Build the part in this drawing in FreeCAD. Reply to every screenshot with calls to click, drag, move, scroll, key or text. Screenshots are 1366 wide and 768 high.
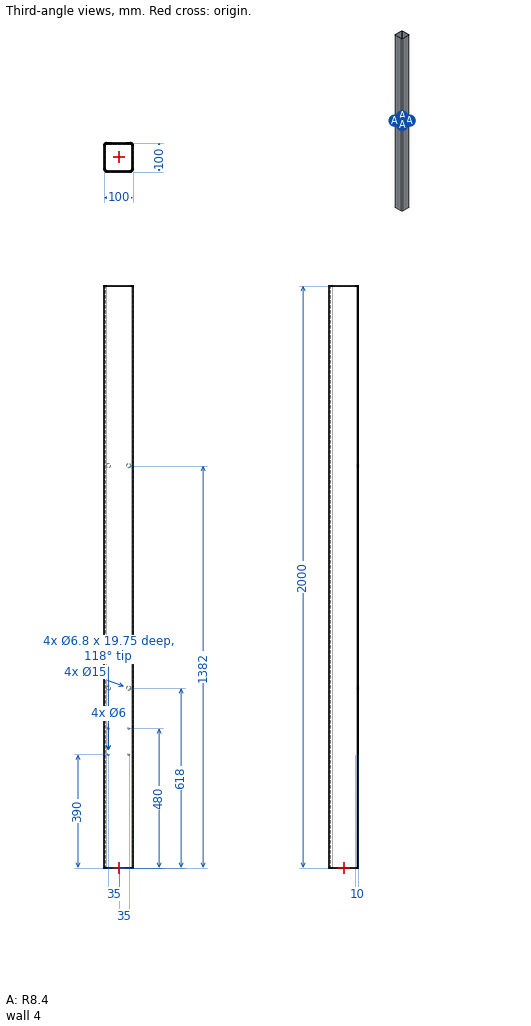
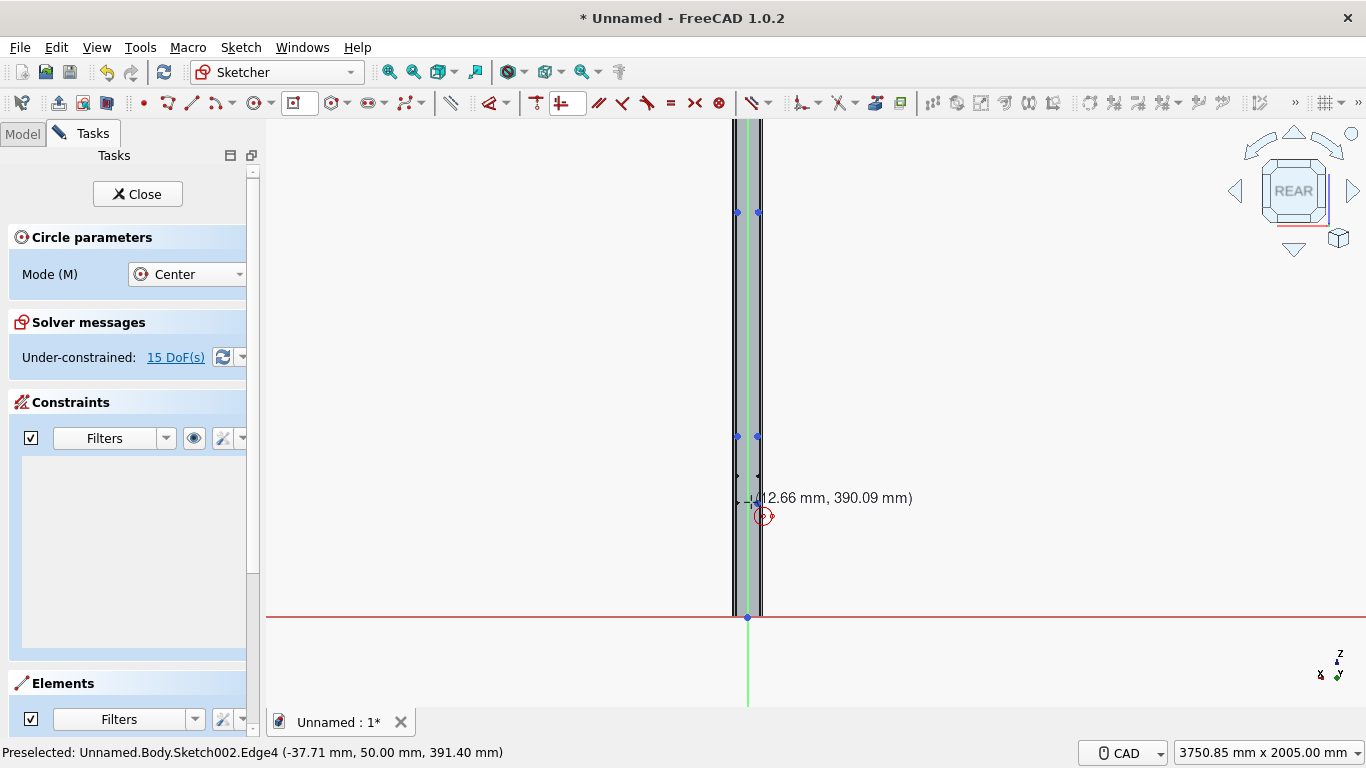
scroll(737, 503, up, 3)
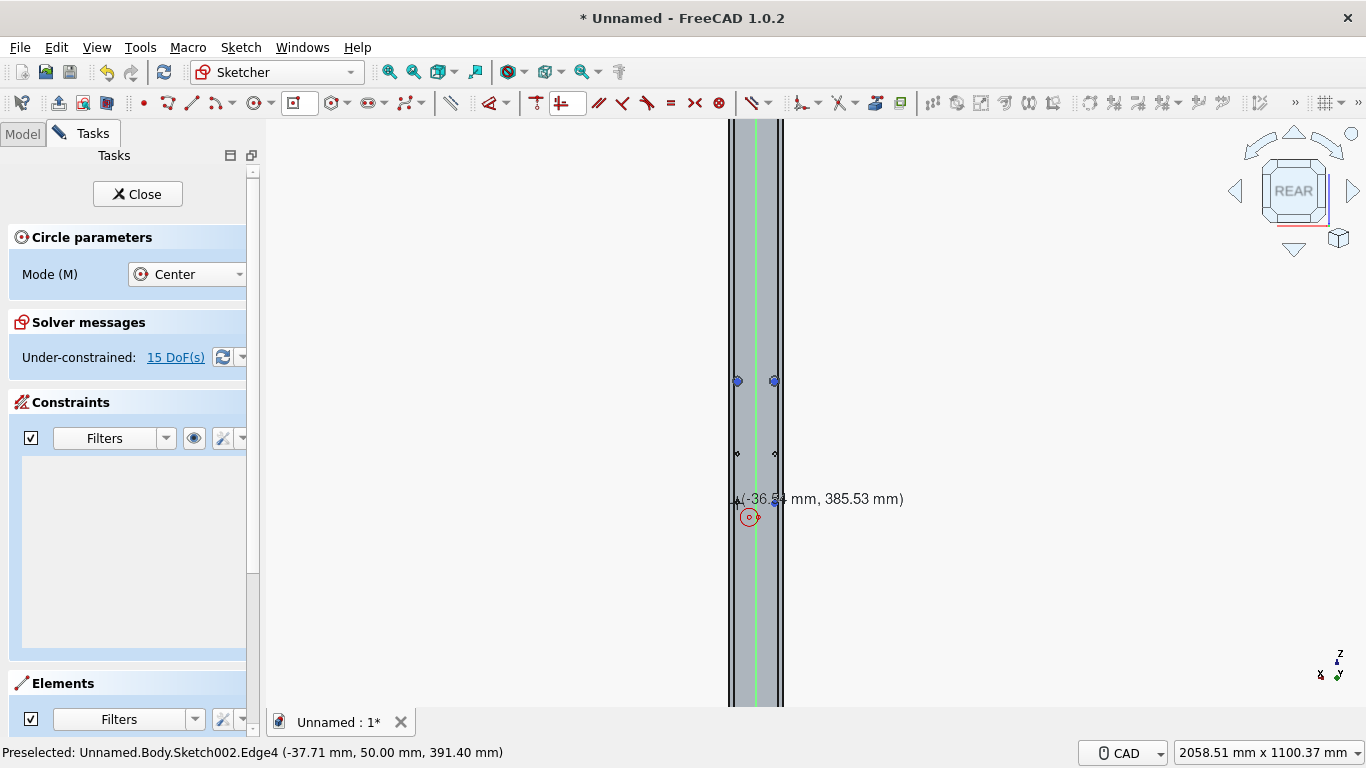
click(737, 502)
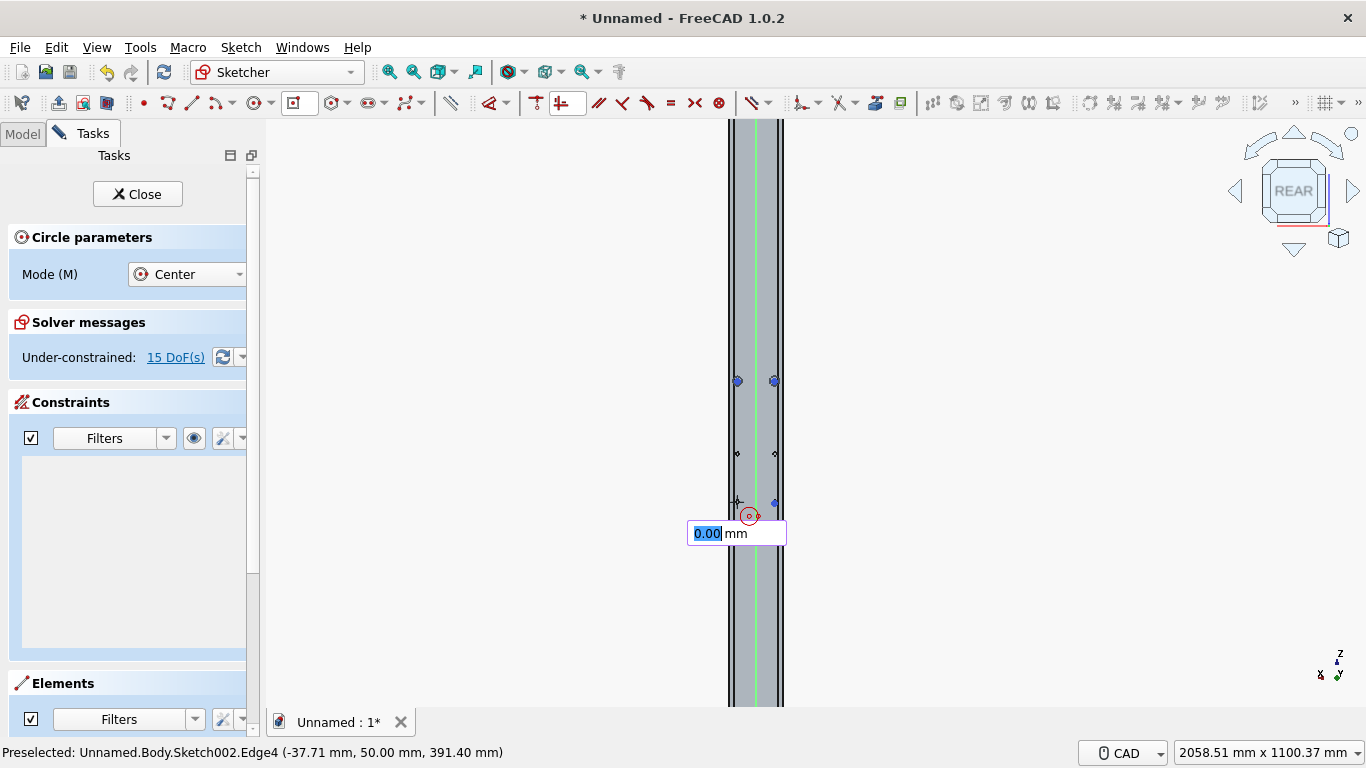
scroll(739, 501, up, 12)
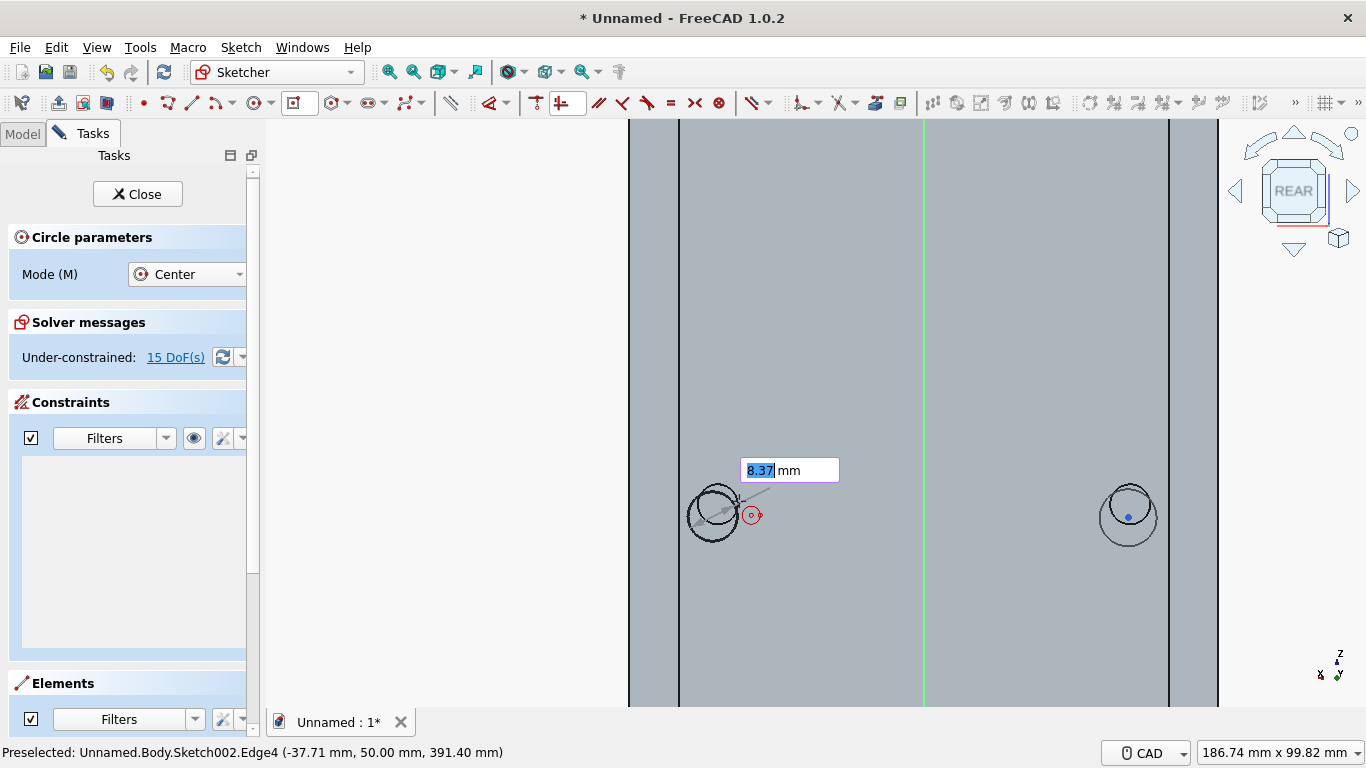
click(730, 492)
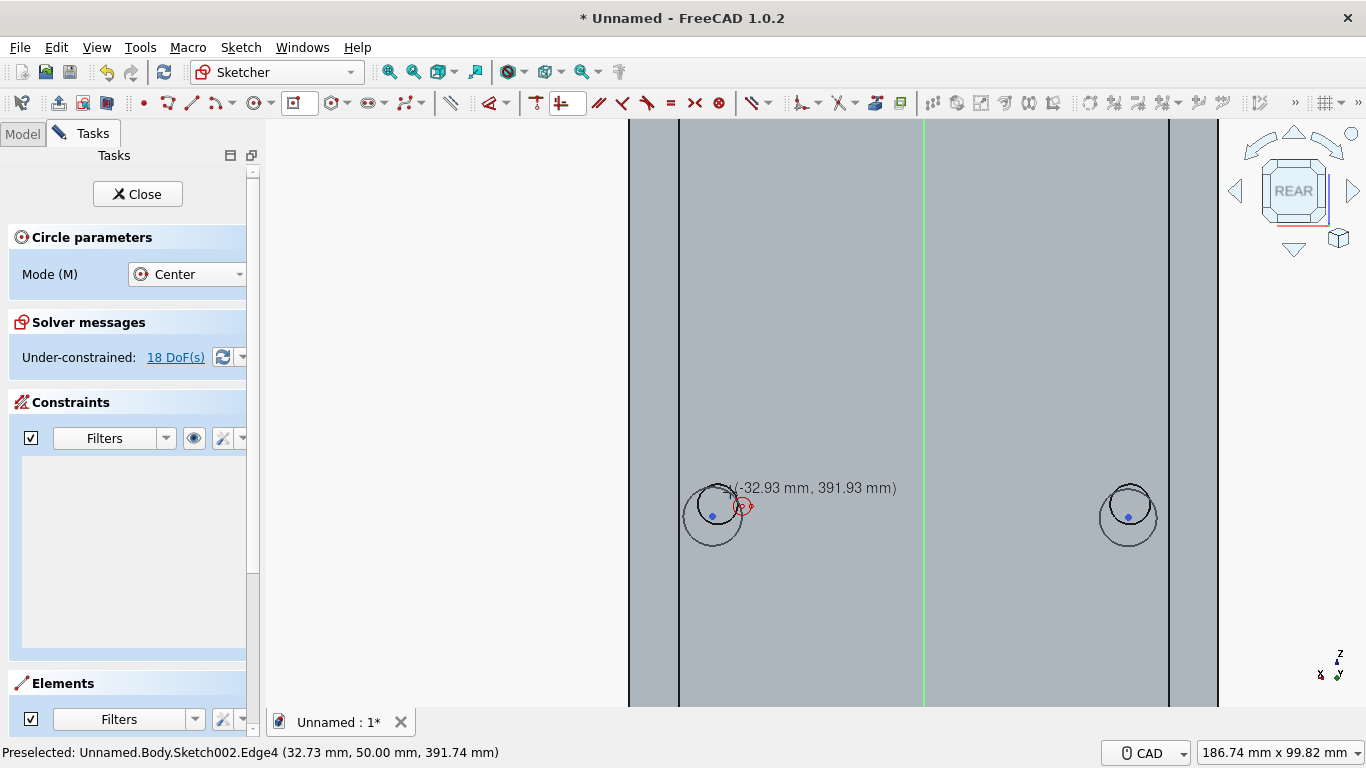
scroll(738, 502, down, 15)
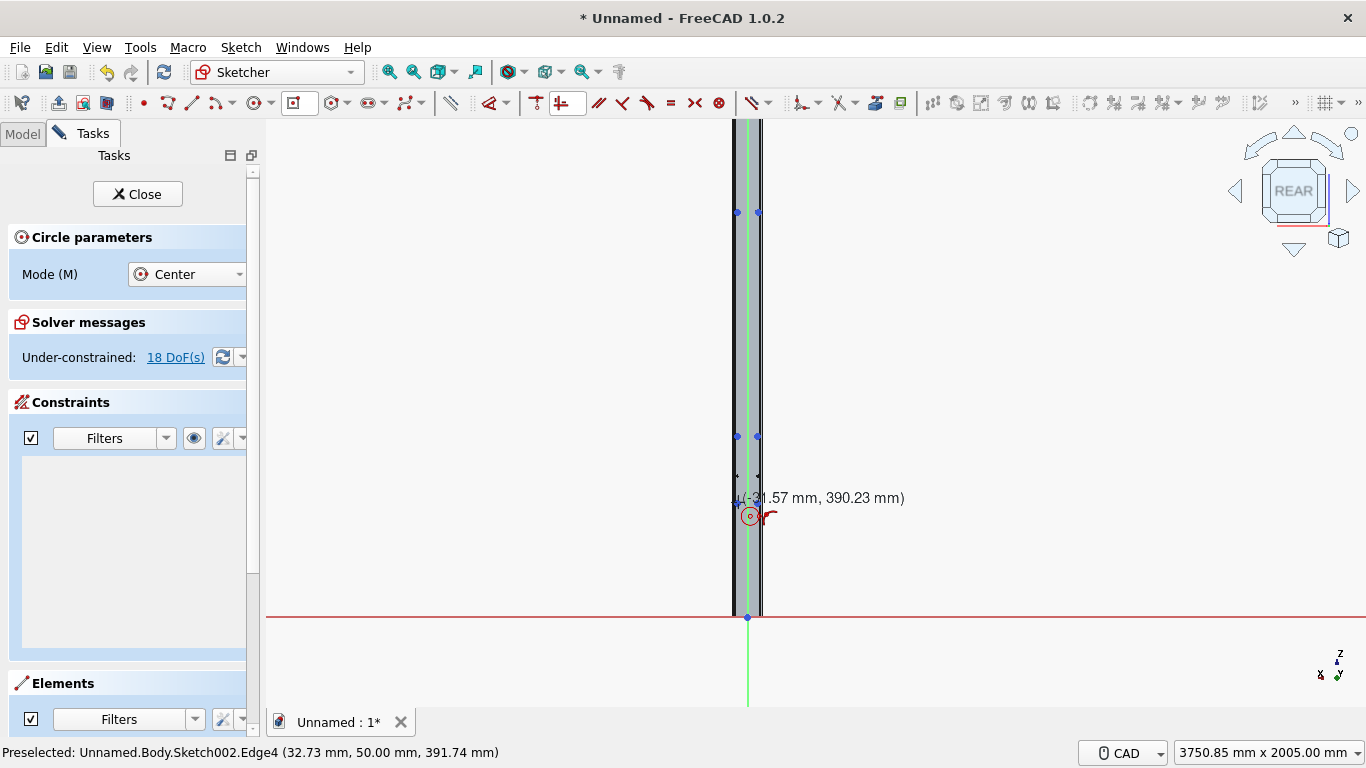
scroll(737, 476, up, 17)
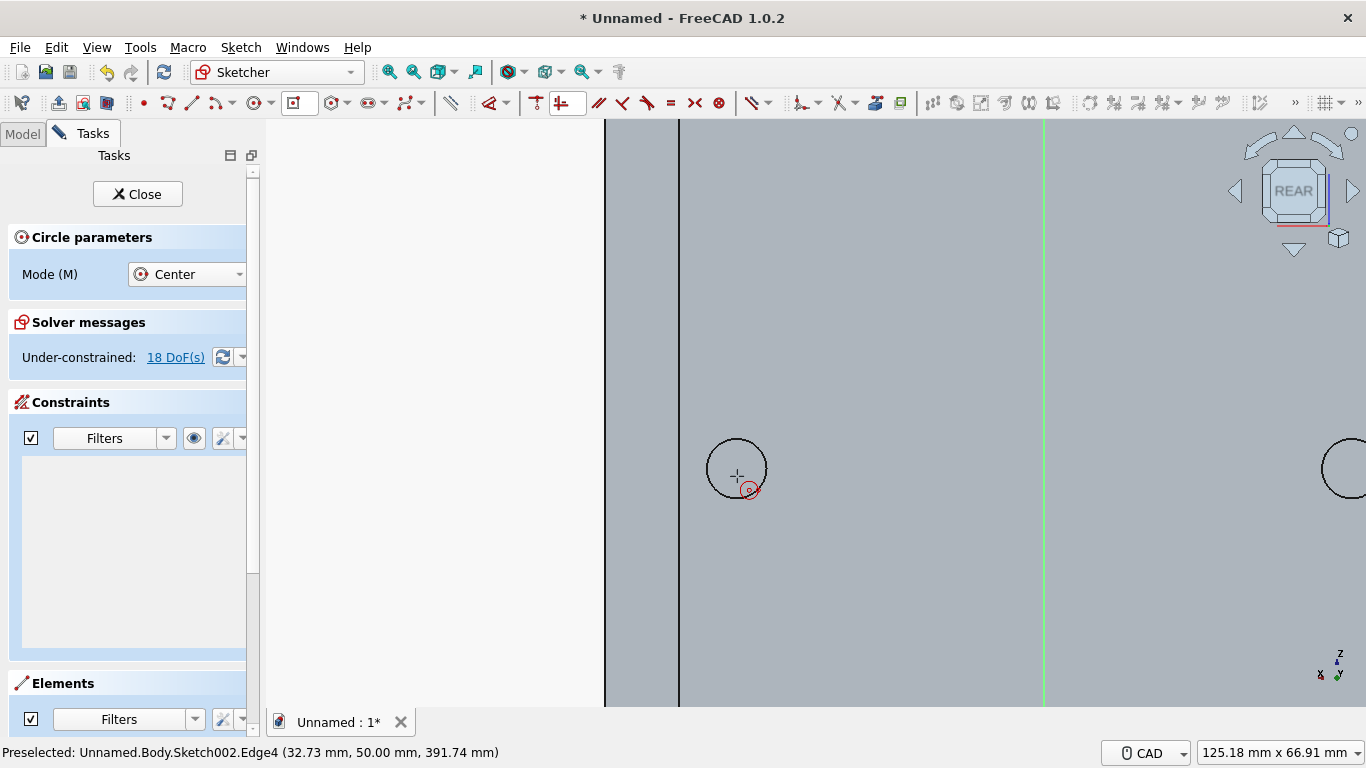
scroll(737, 476, down, 17)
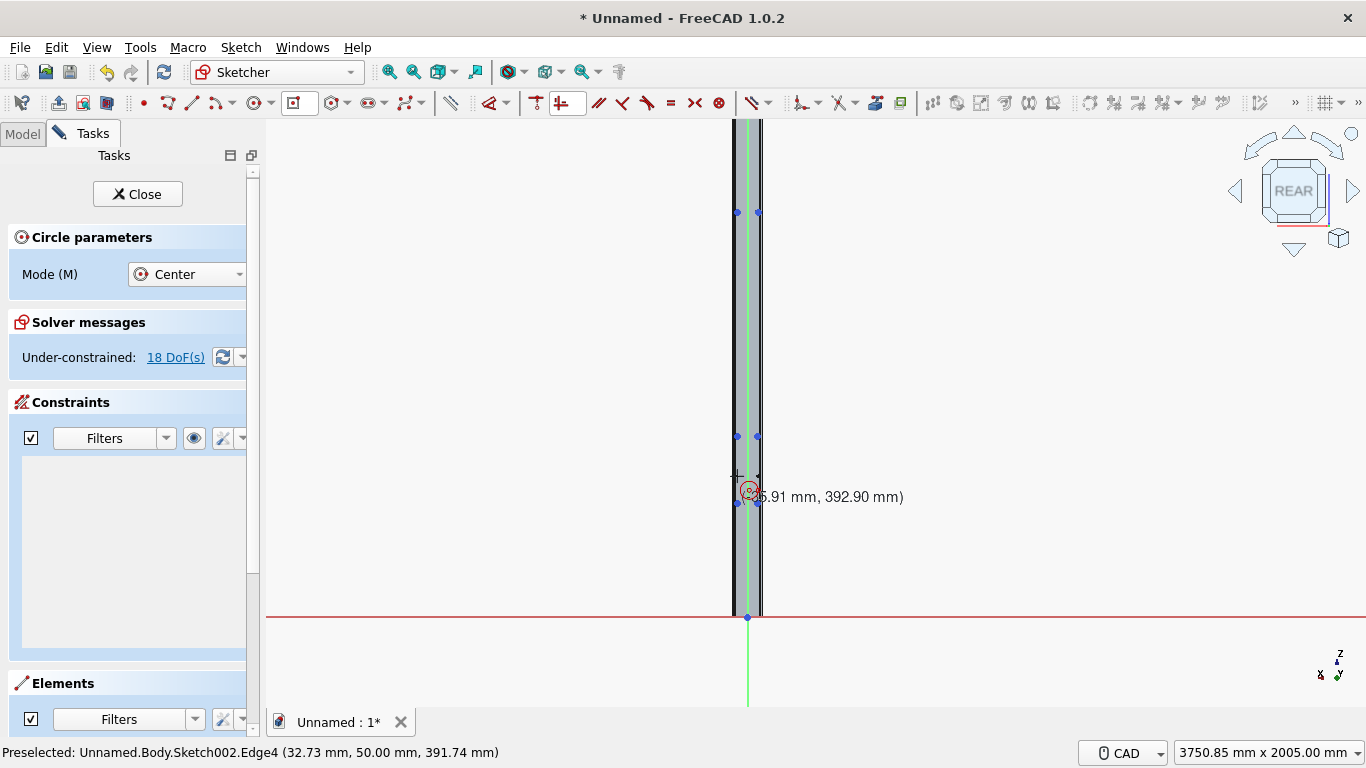
scroll(737, 476, up, 3)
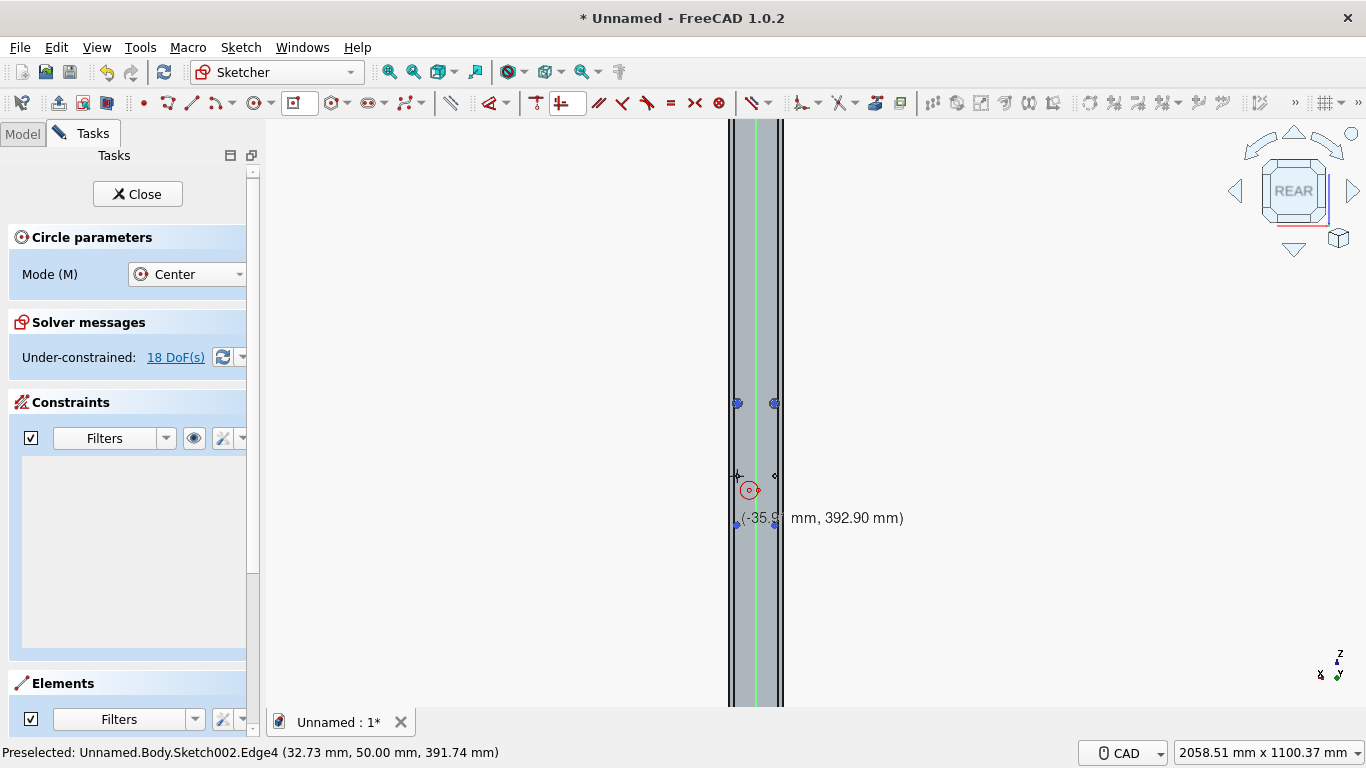
click(737, 476)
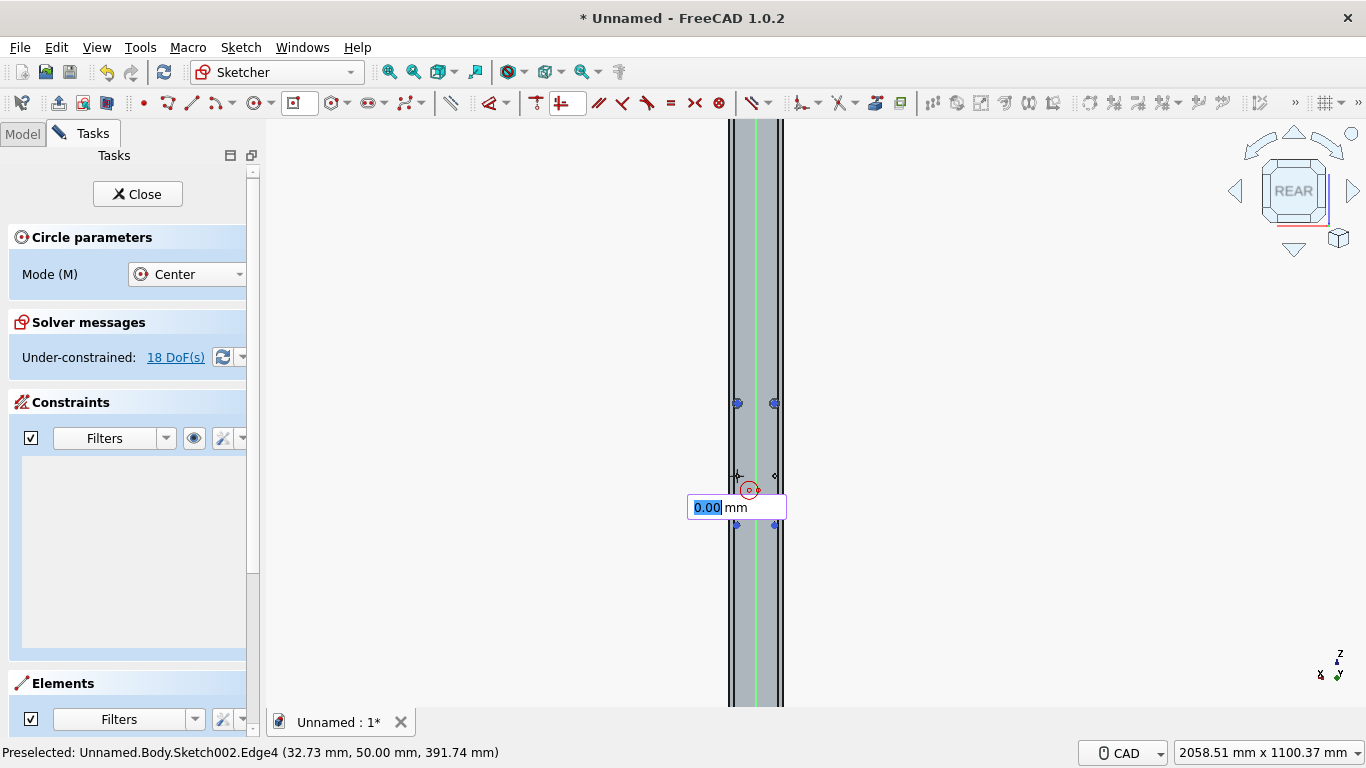
scroll(739, 475, up, 12)